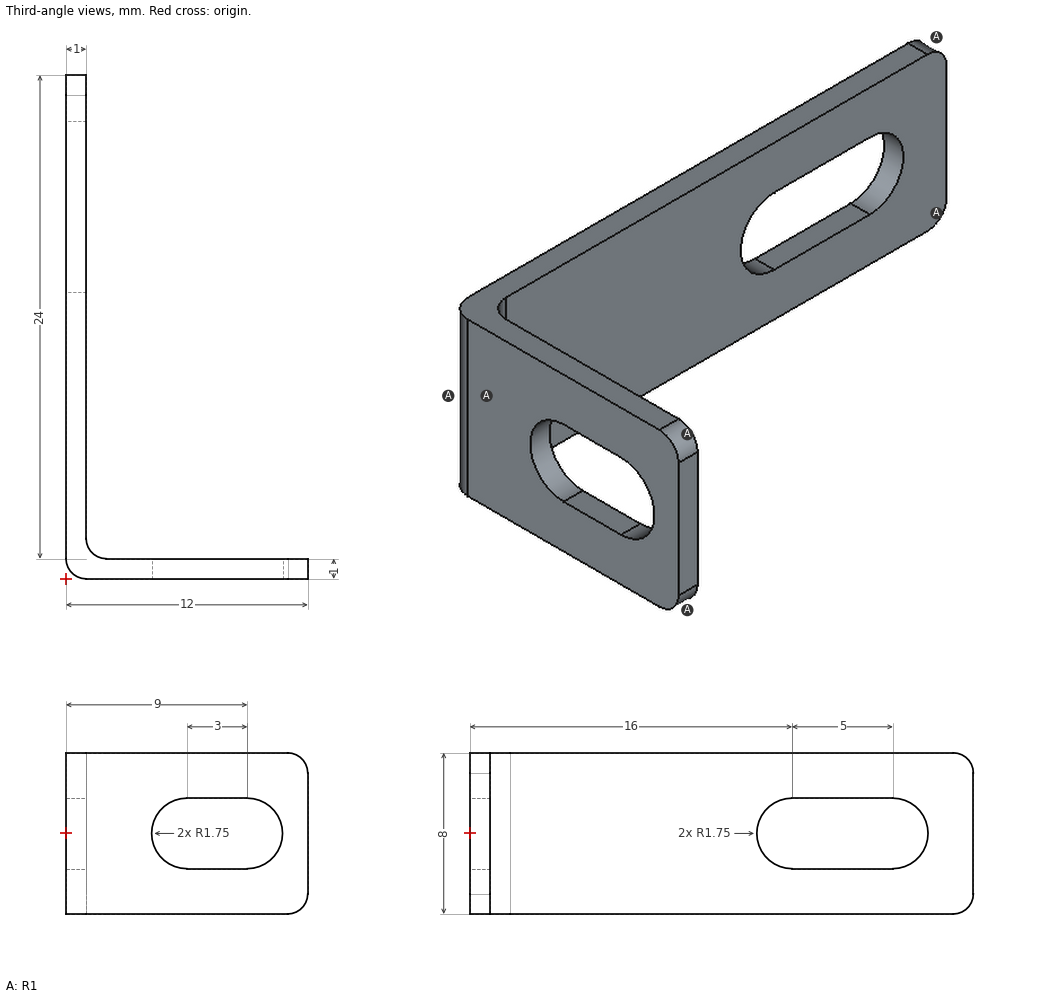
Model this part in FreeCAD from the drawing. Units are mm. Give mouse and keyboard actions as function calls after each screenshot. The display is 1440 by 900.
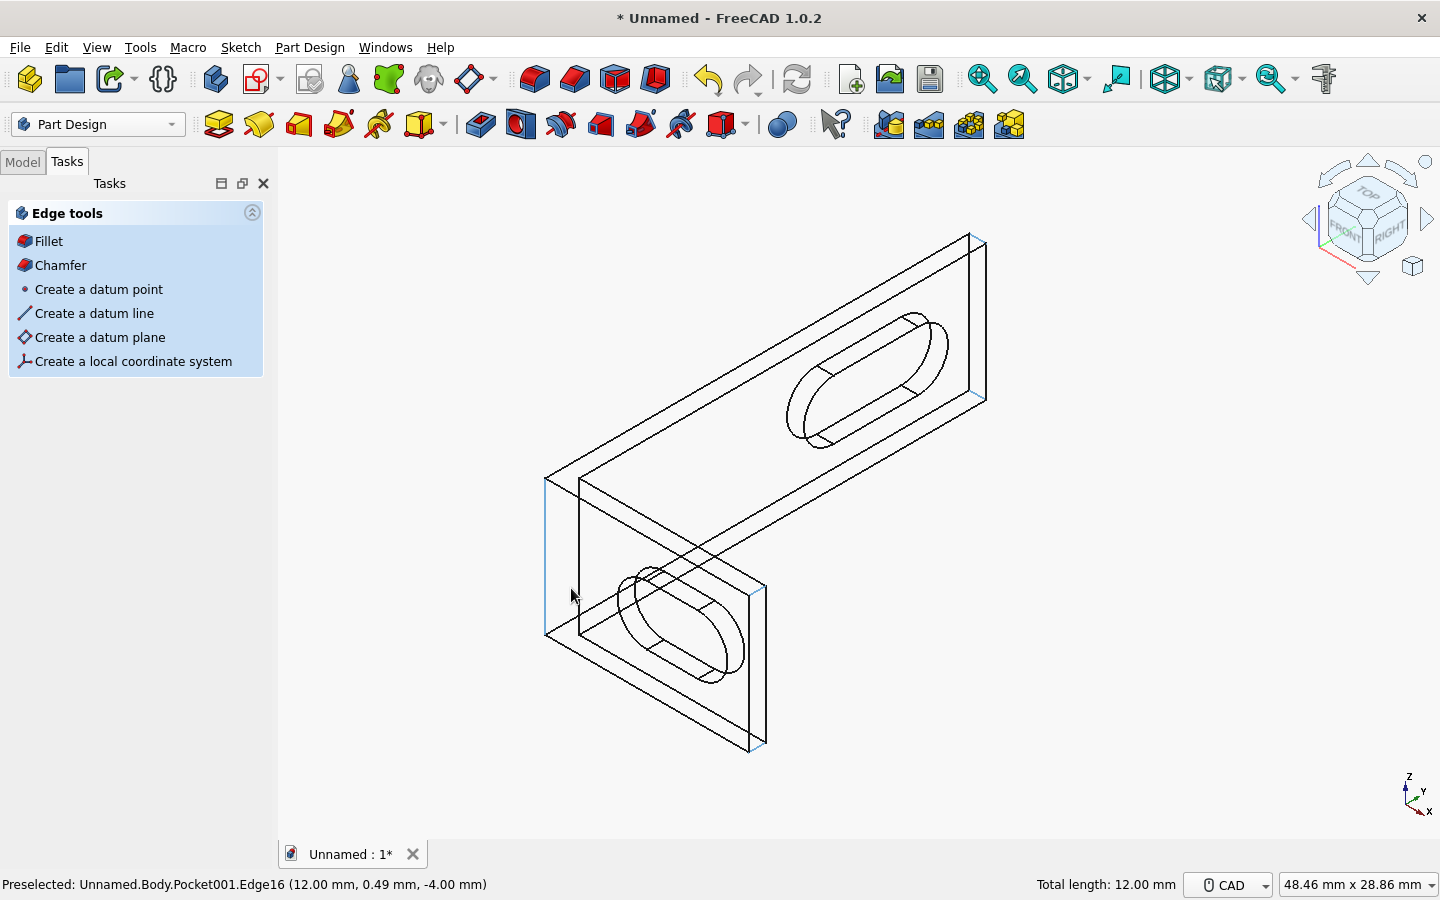
click(579, 556, ctrl)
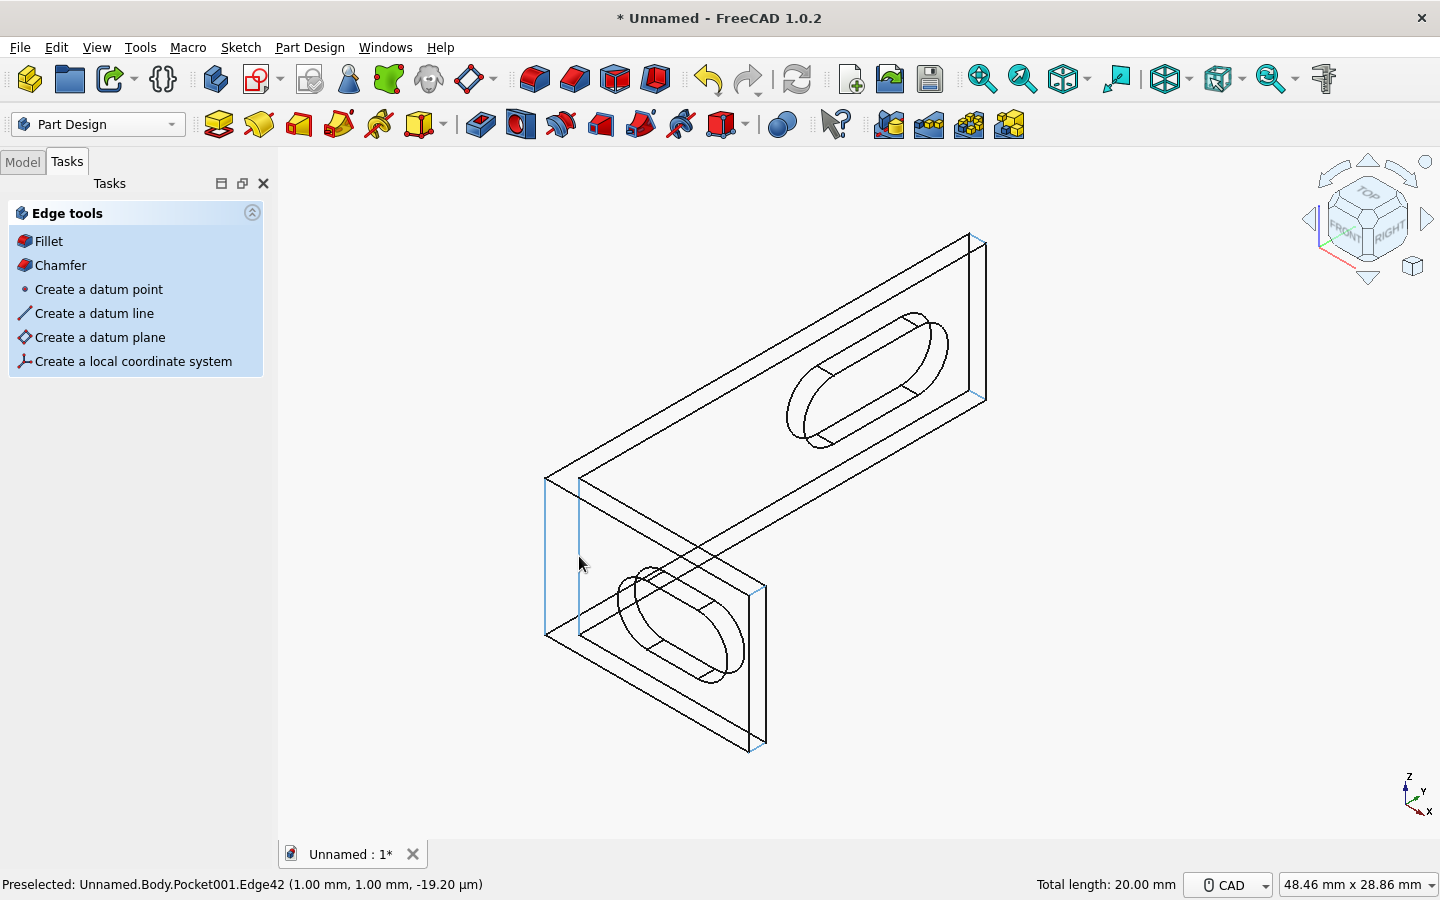
key(v)
key(1)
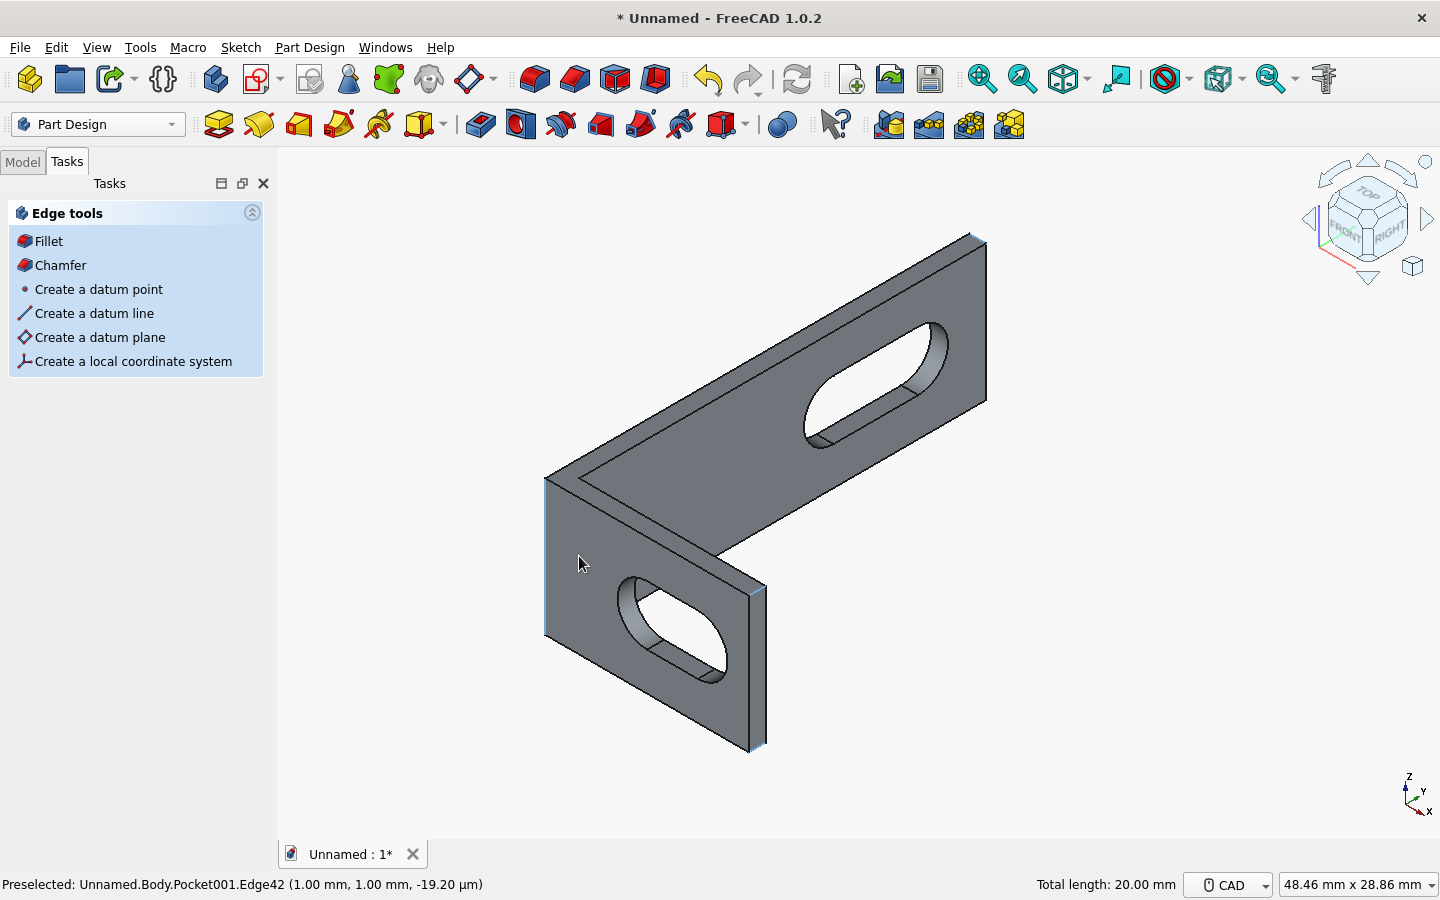
click(536, 80)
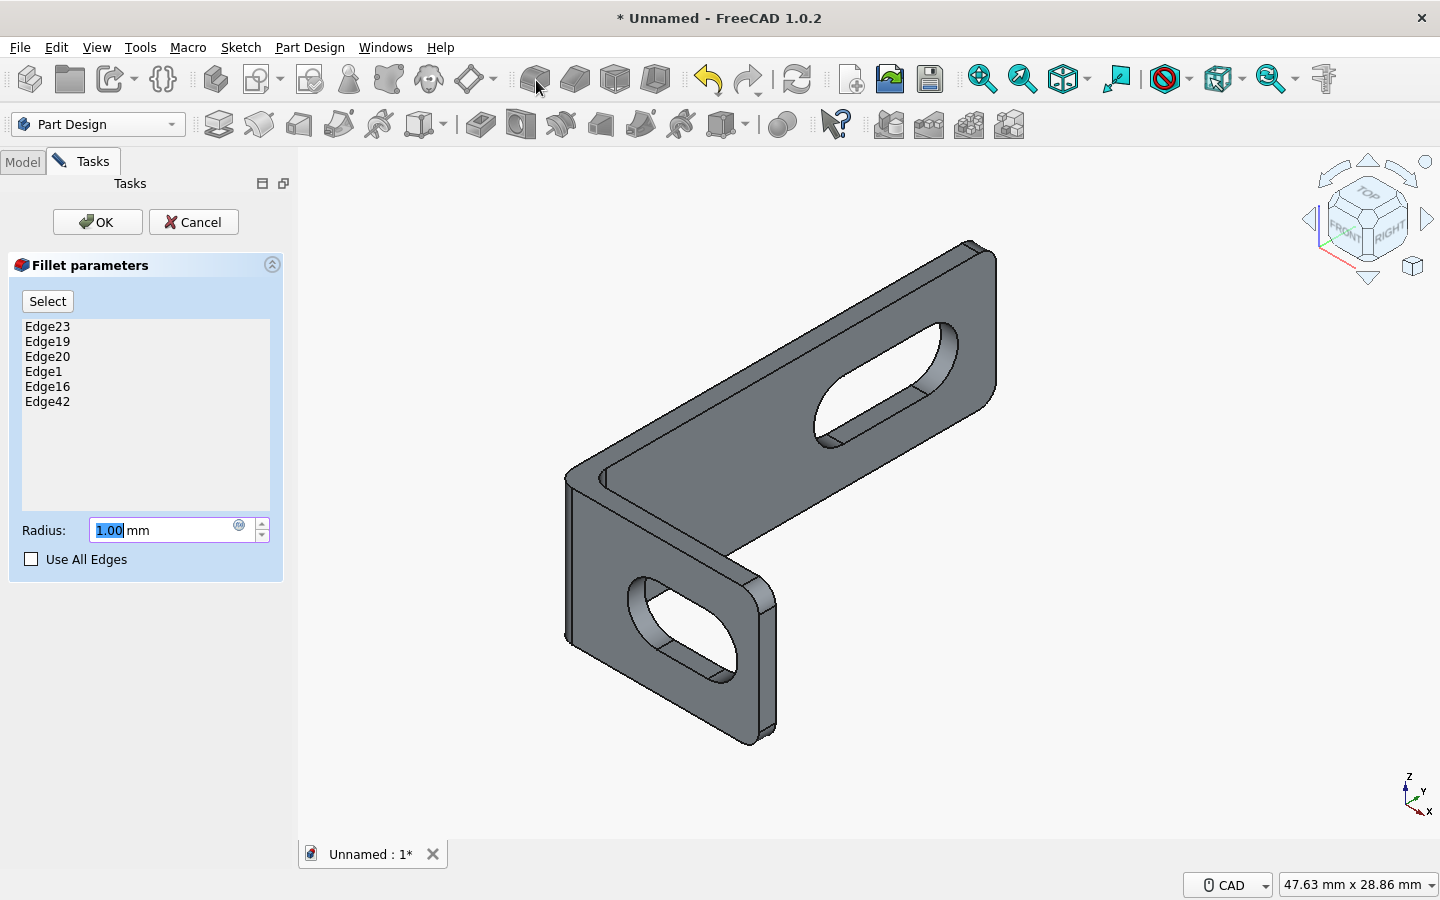
text(1)
key(Tab)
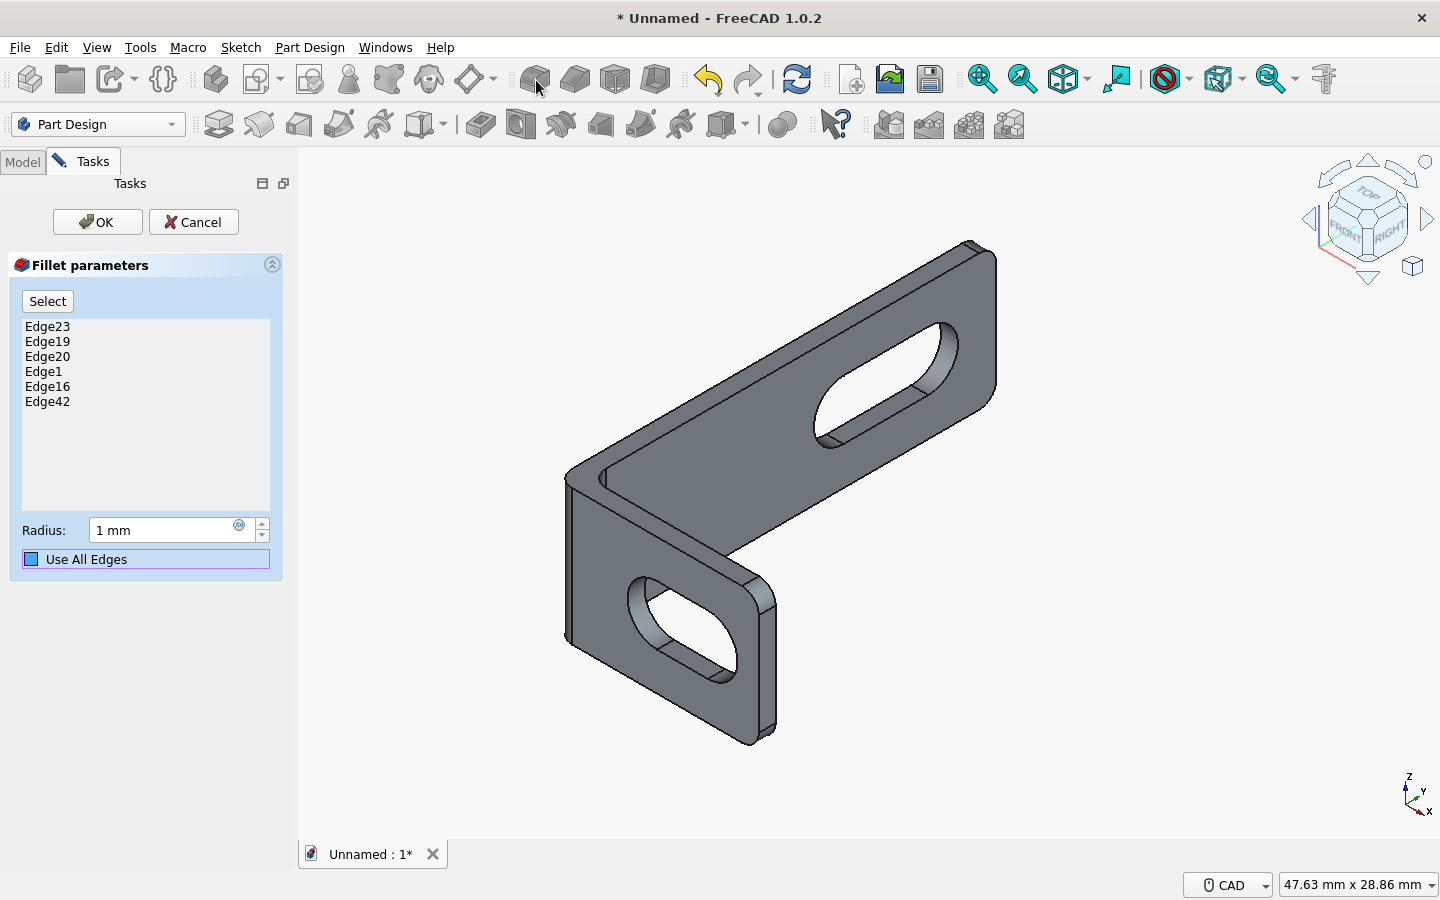
click(98, 222)